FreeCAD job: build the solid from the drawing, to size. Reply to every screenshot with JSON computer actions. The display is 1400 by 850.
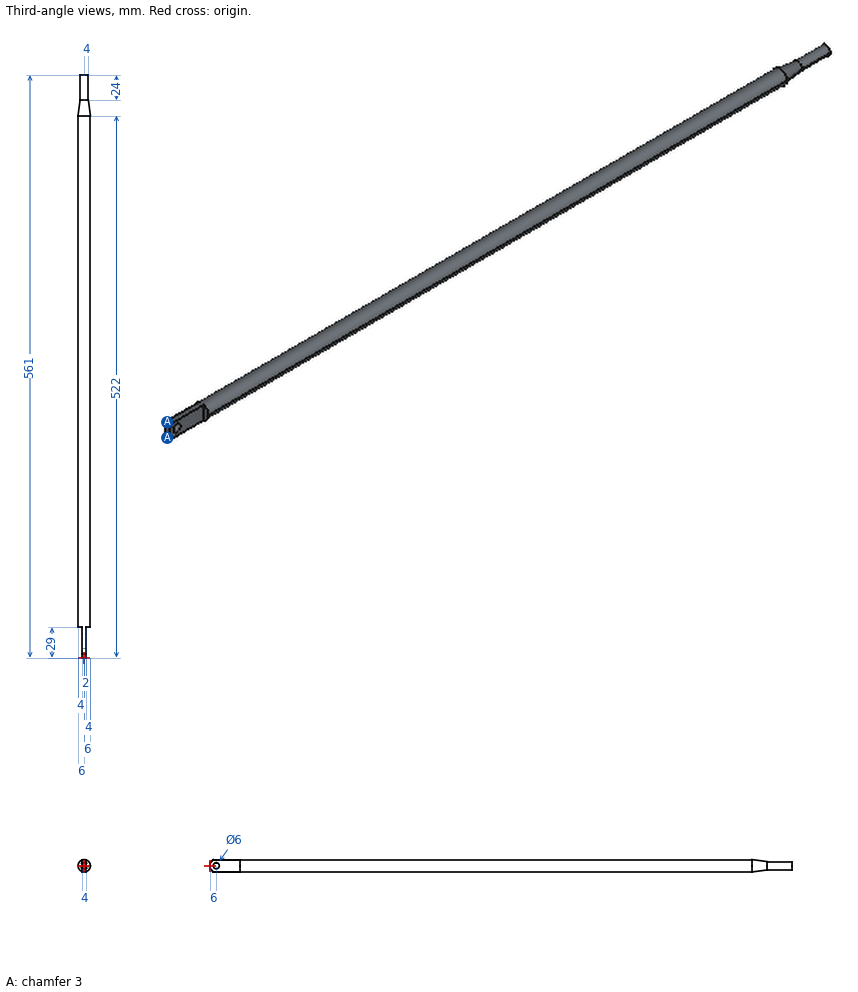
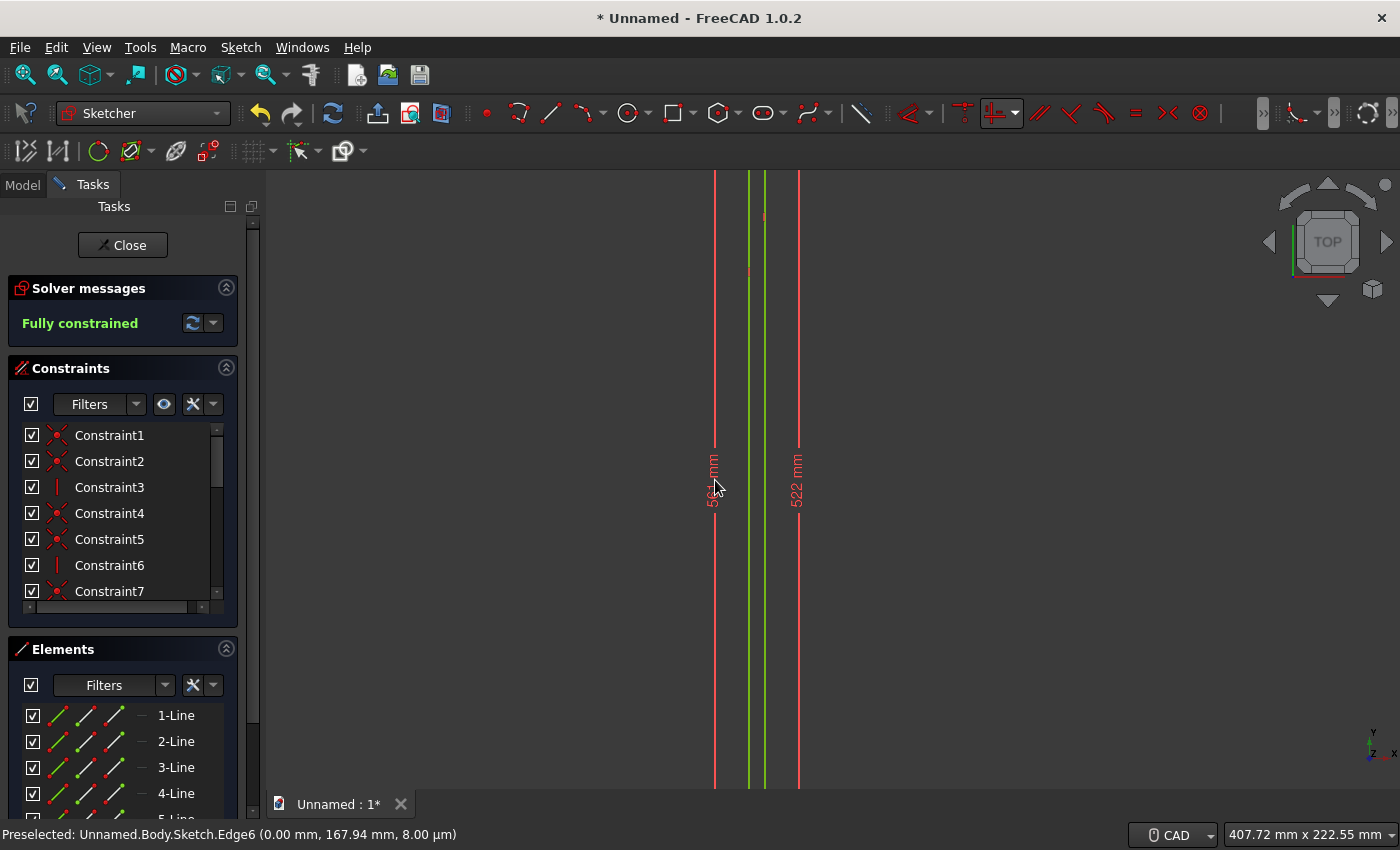
{"action": "left_click", "coordinate": [123, 245]}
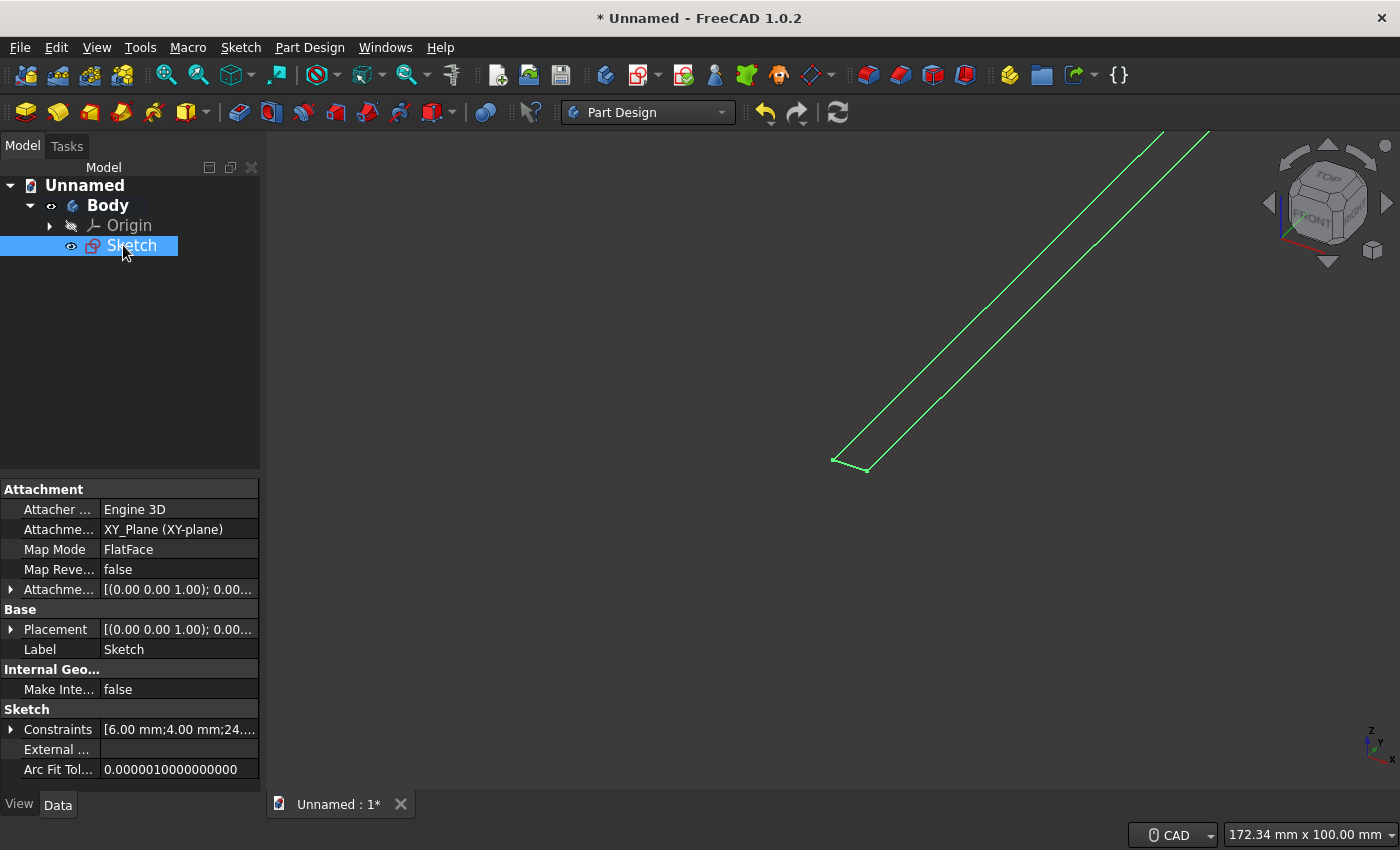
{"action": "left_click", "coordinate": [58, 112]}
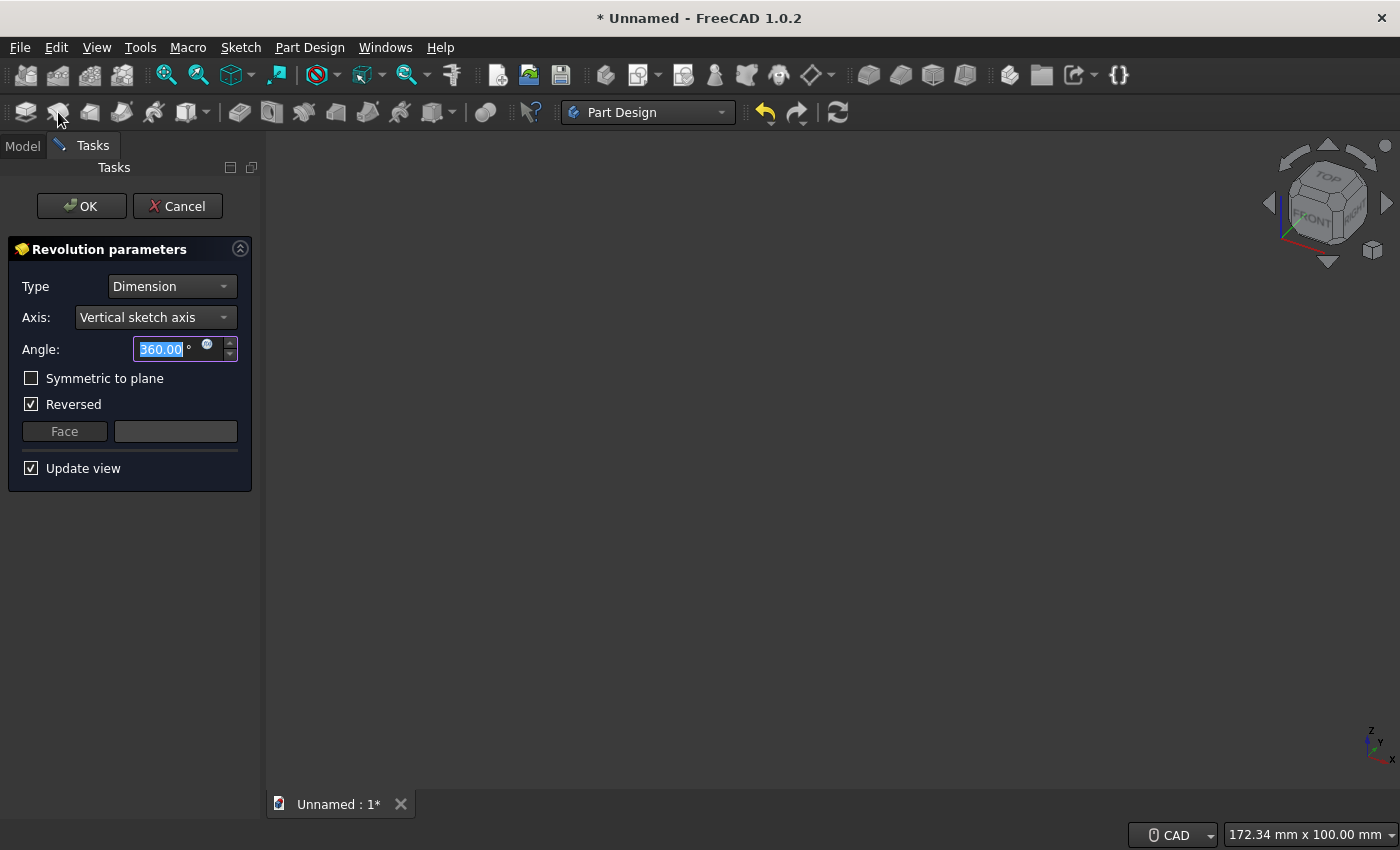
{"action": "left_click", "coordinate": [82, 206]}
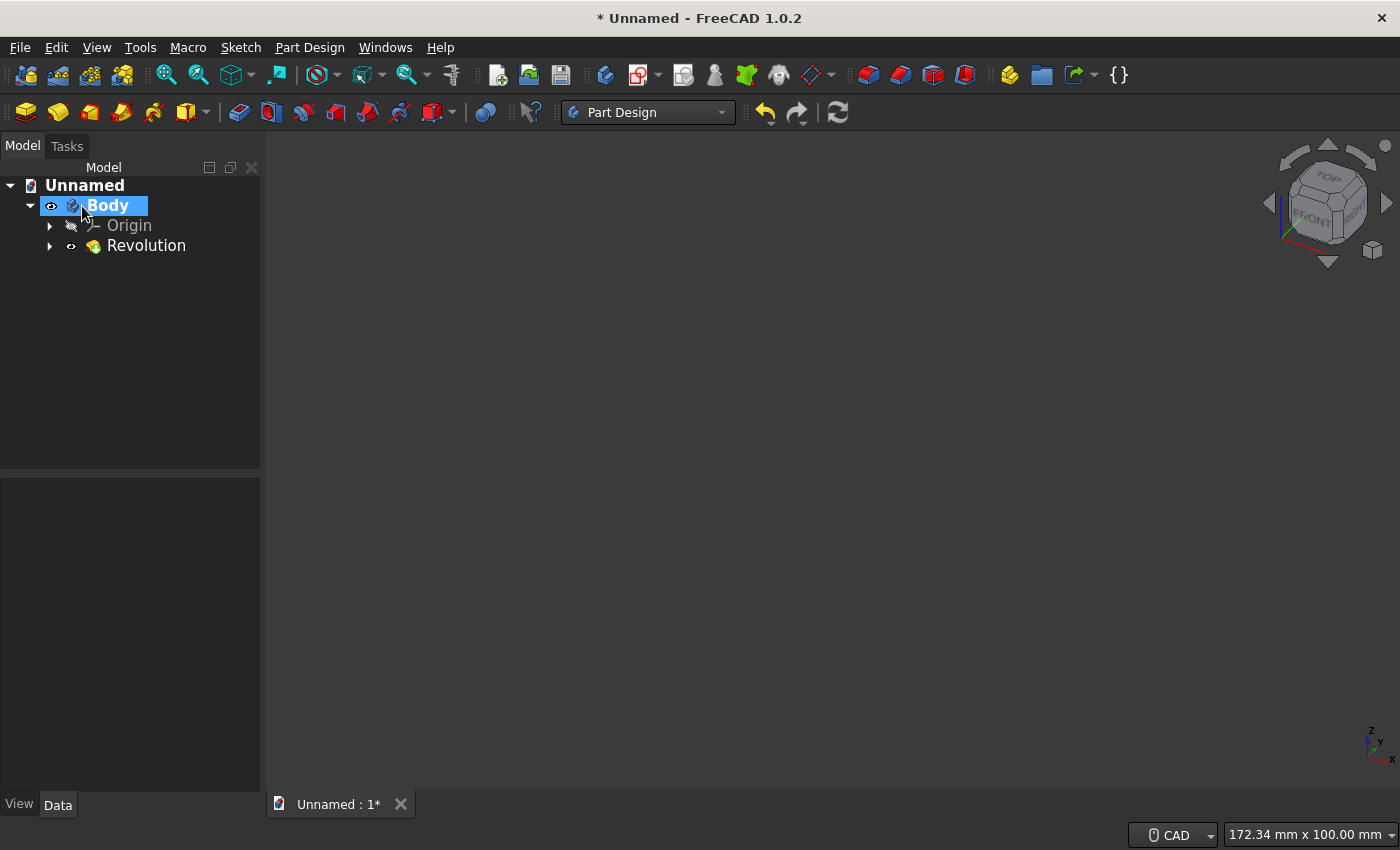
{"action": "left_click", "coordinate": [168, 76]}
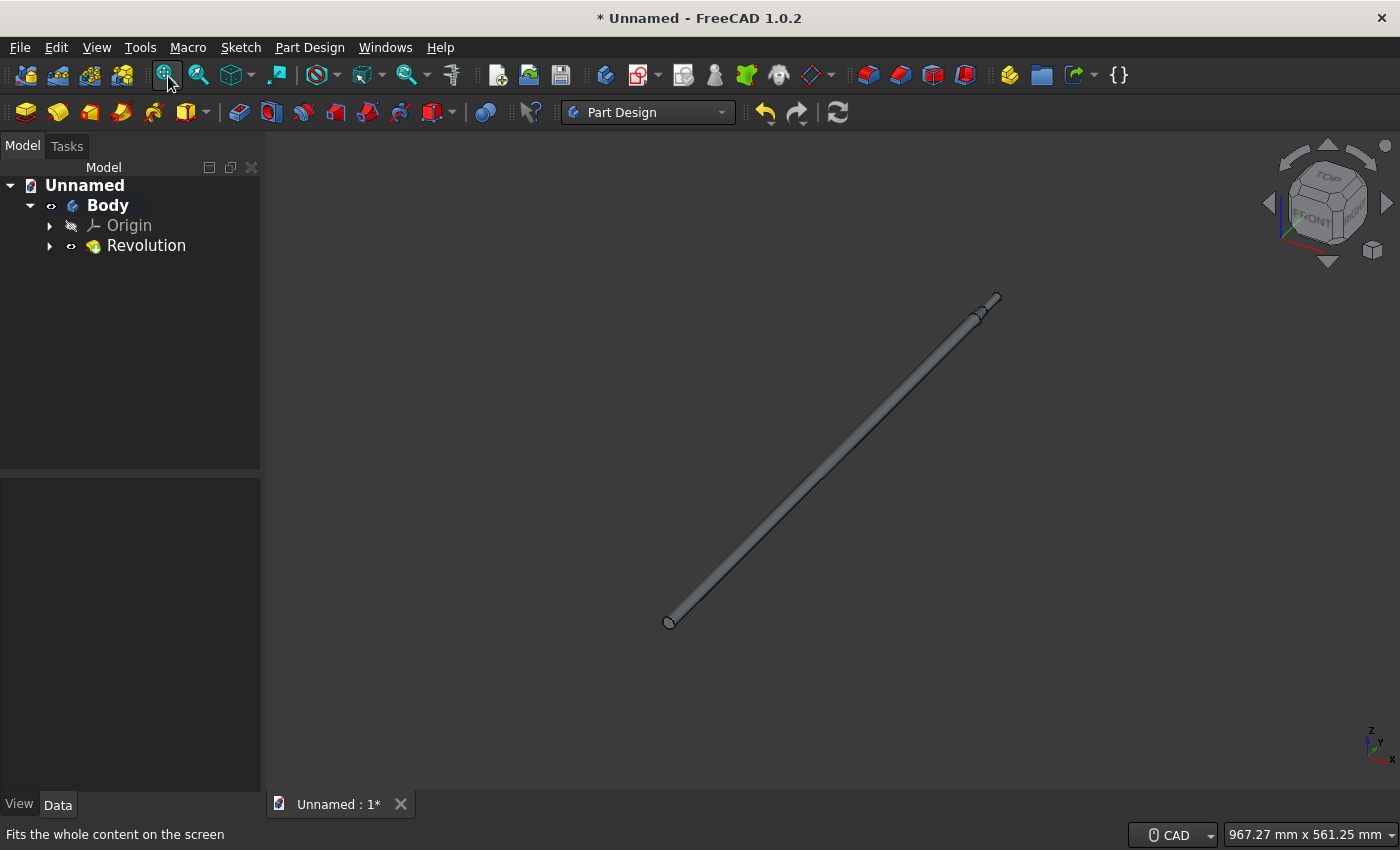
{"action": "left_click", "coordinate": [638, 76]}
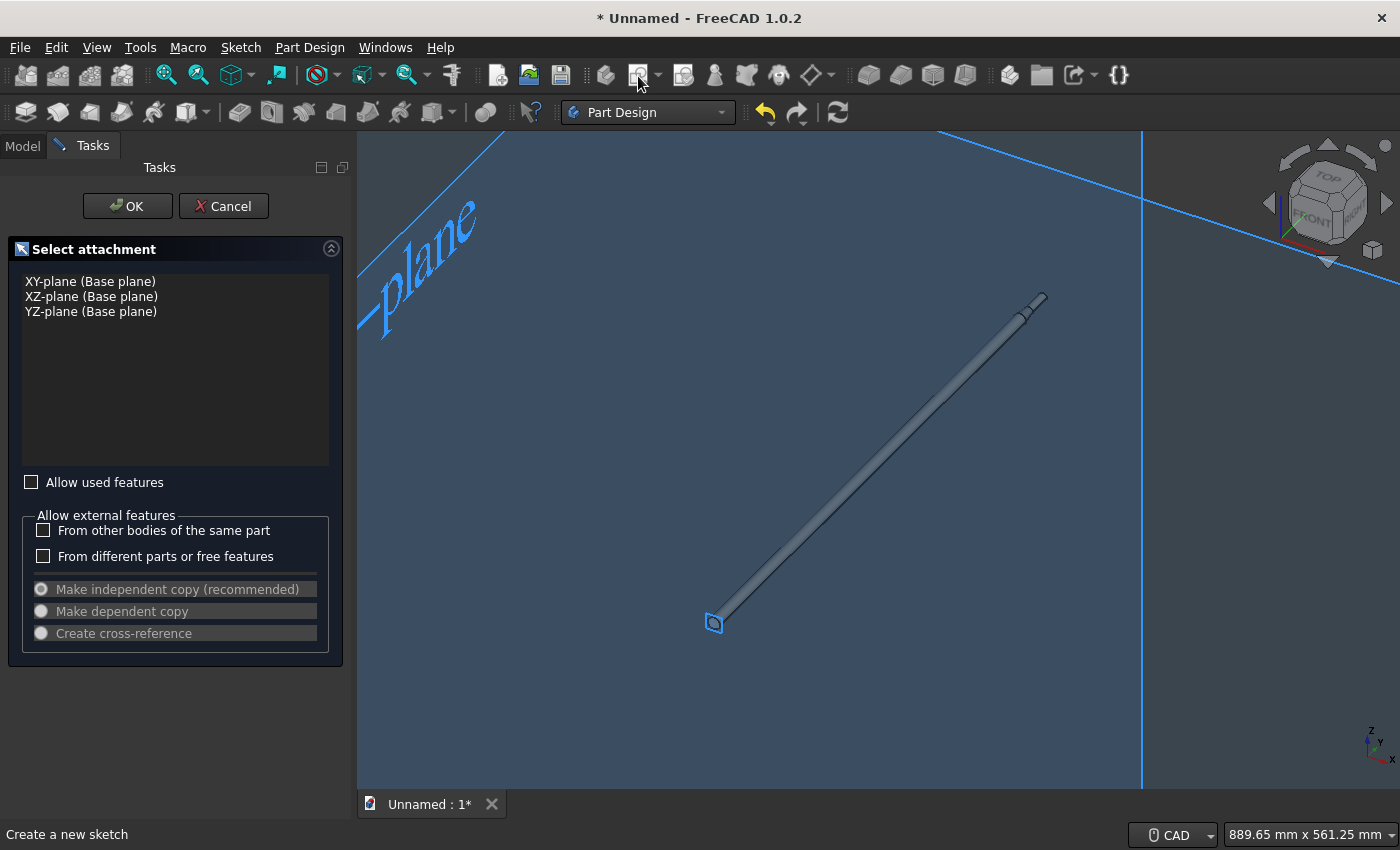
{"action": "left_click", "coordinate": [82, 282]}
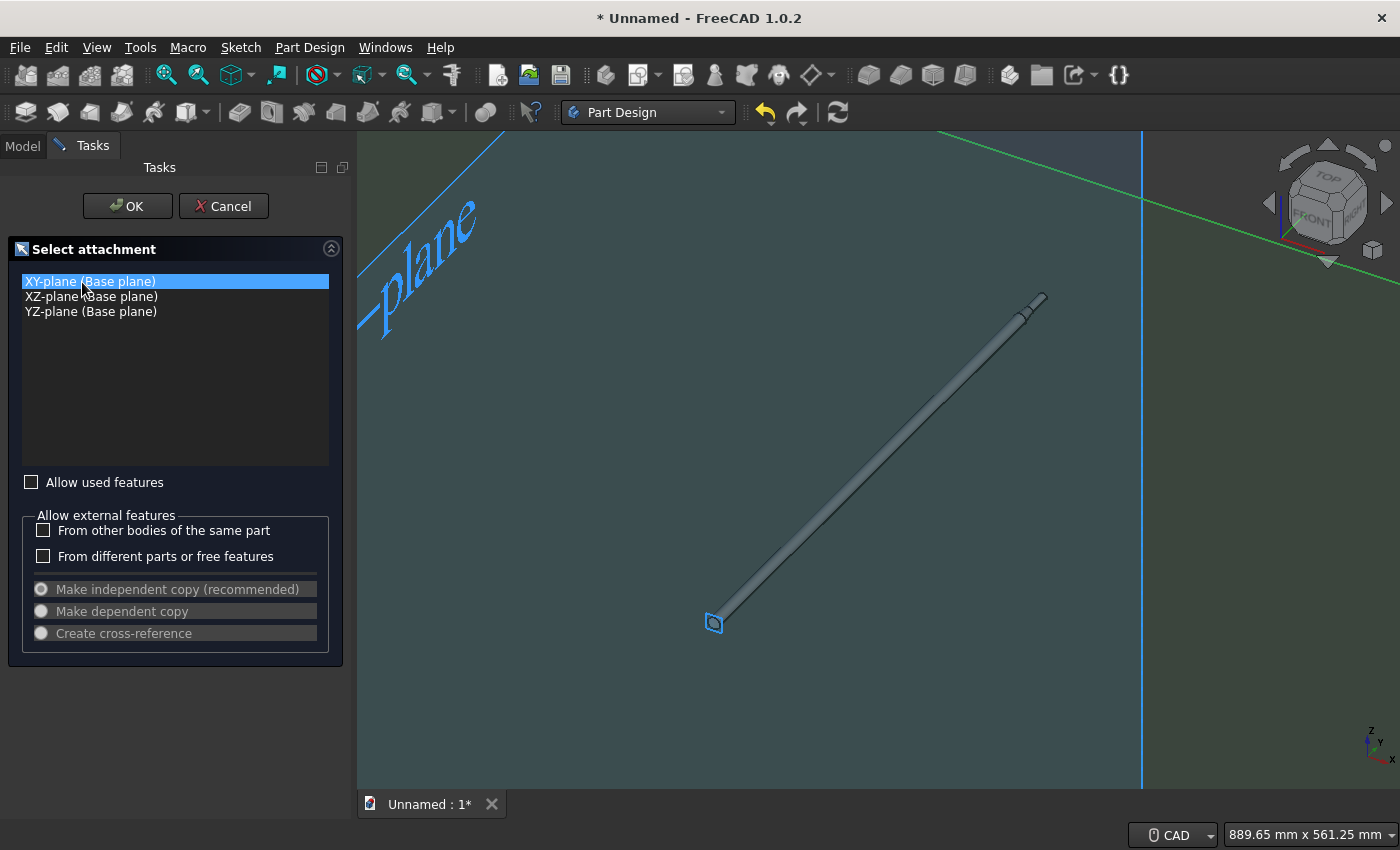
{"action": "left_click", "coordinate": [128, 206]}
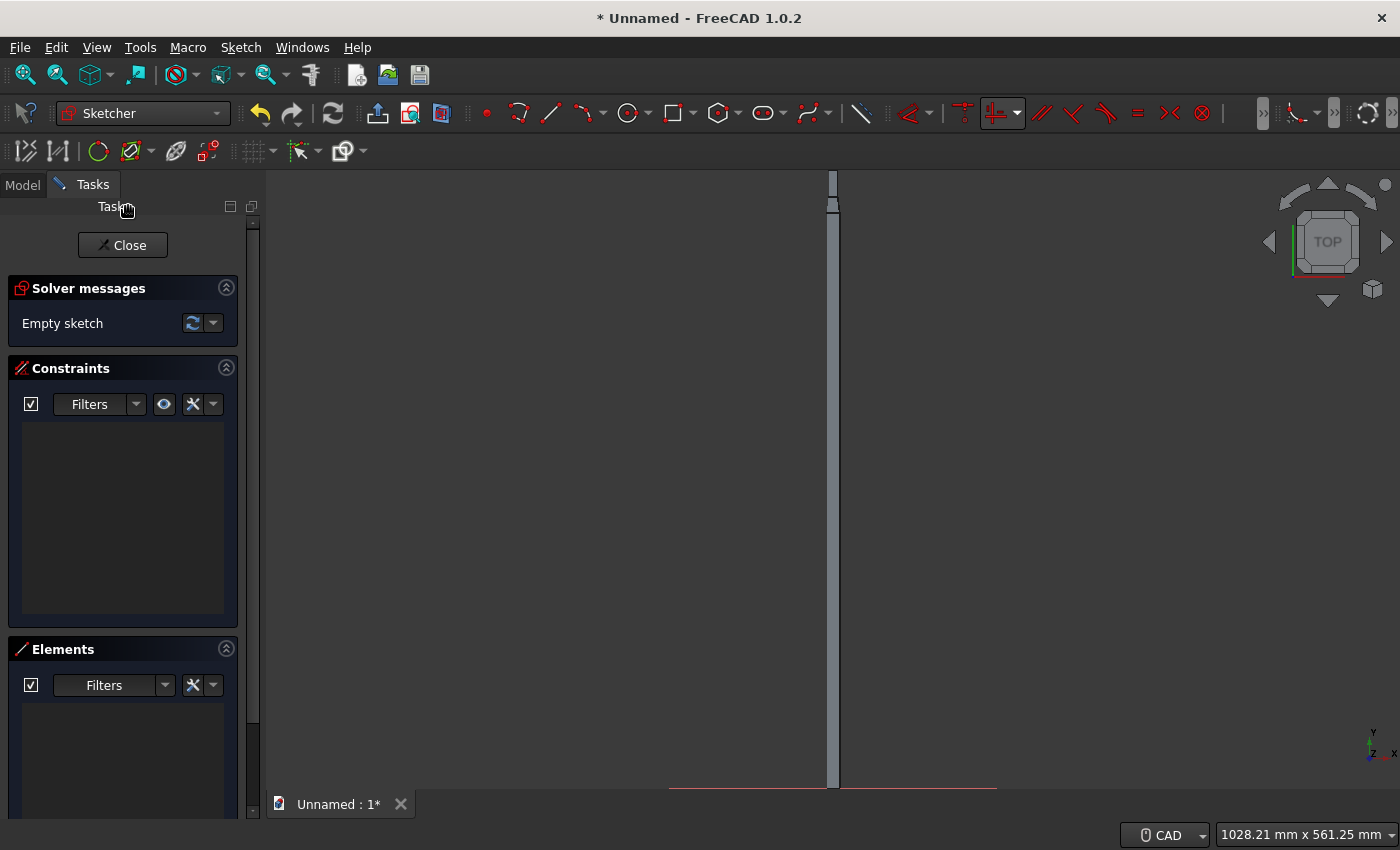
{"action": "left_click", "coordinate": [442, 114]}